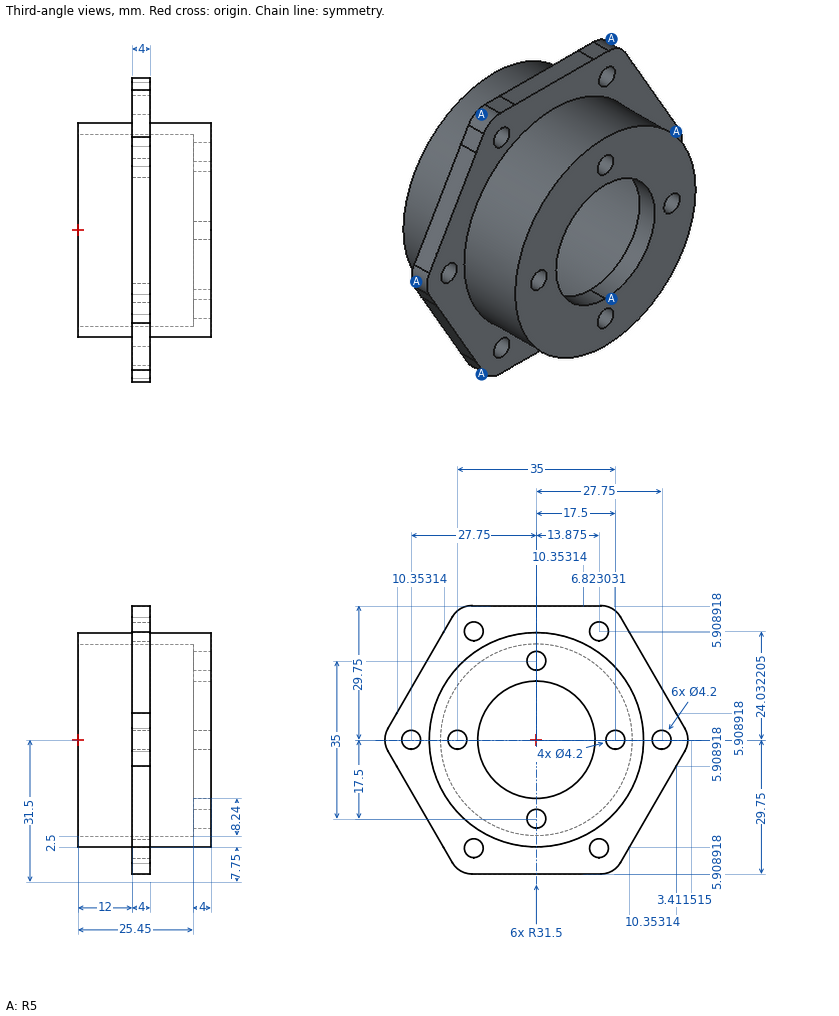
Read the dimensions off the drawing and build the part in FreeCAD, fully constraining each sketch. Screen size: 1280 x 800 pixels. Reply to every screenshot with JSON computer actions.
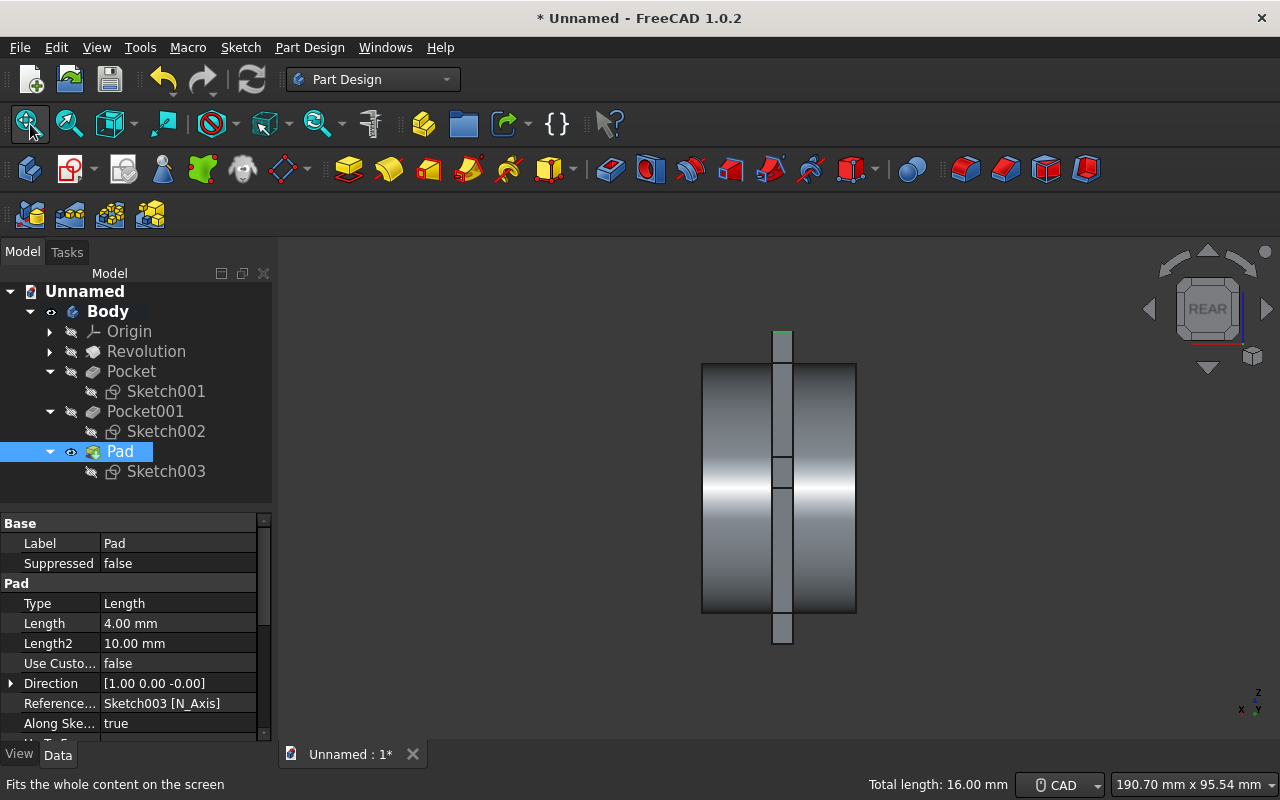
{"action": "left_click", "coordinate": [783, 487], "text": "ctrl"}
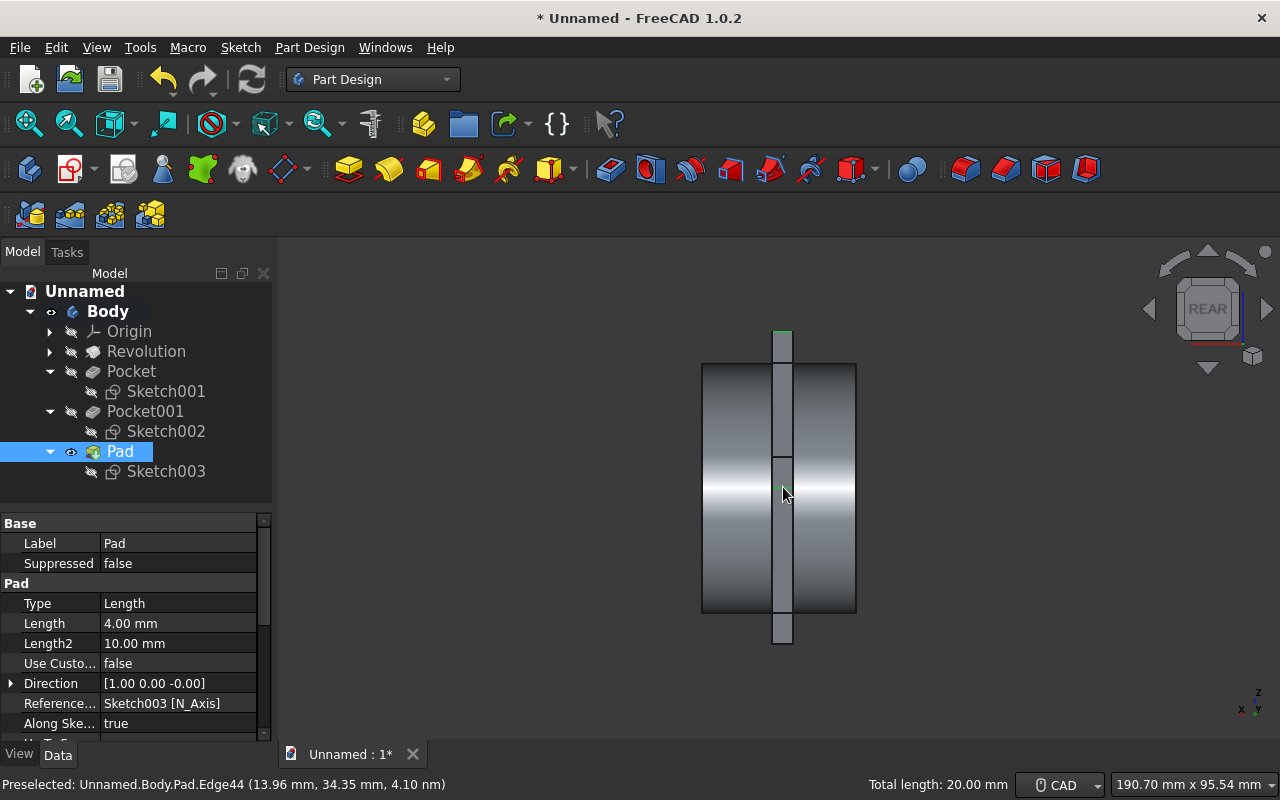
{"action": "scroll", "coordinate": [783, 643], "scroll_direction": "up", "scroll_amount": 4}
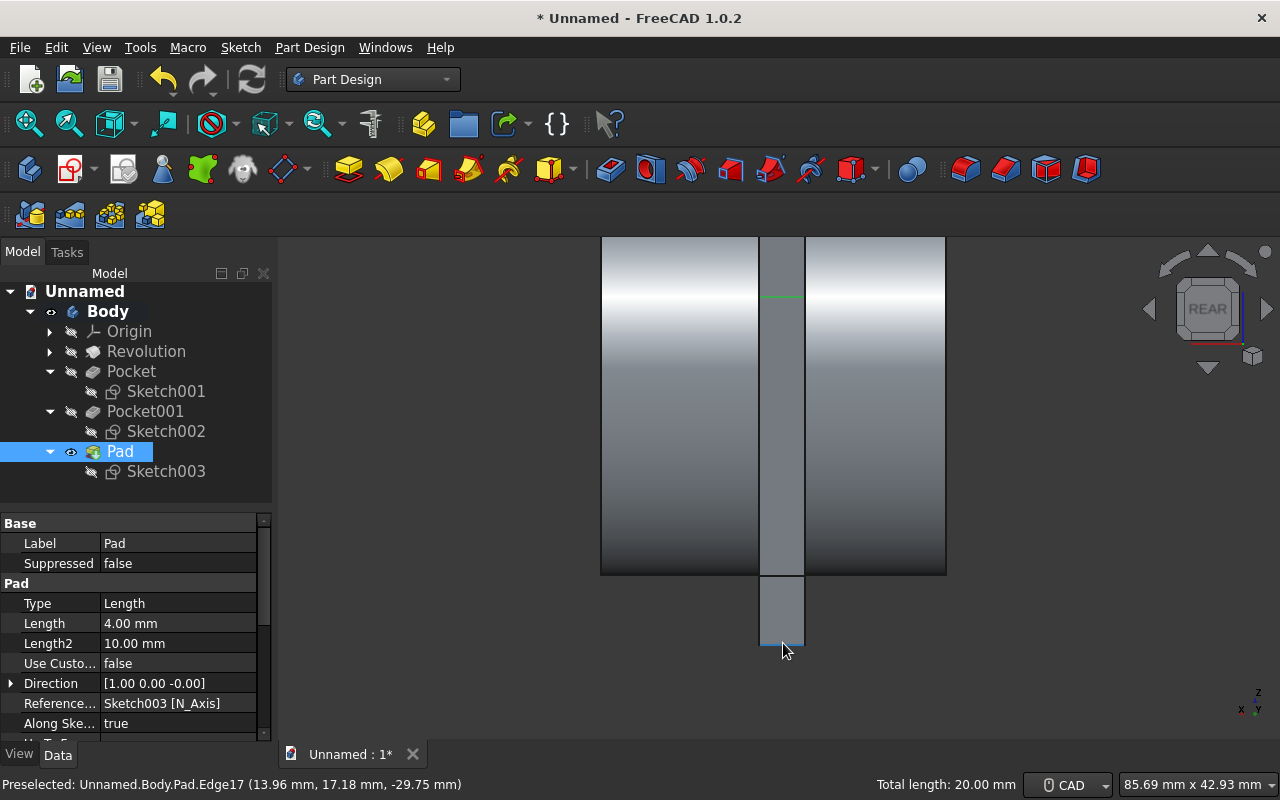
{"action": "key", "text": "v f"}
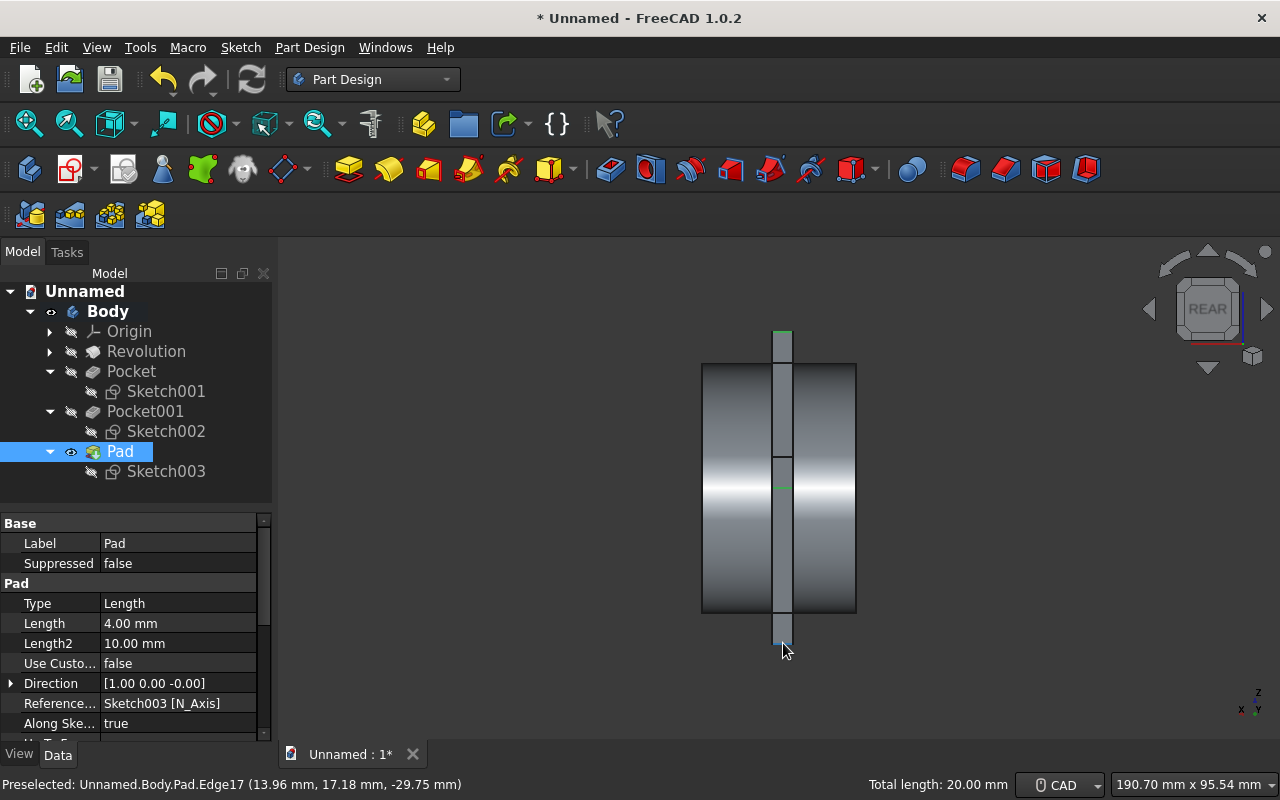
{"action": "key", "text": "6"}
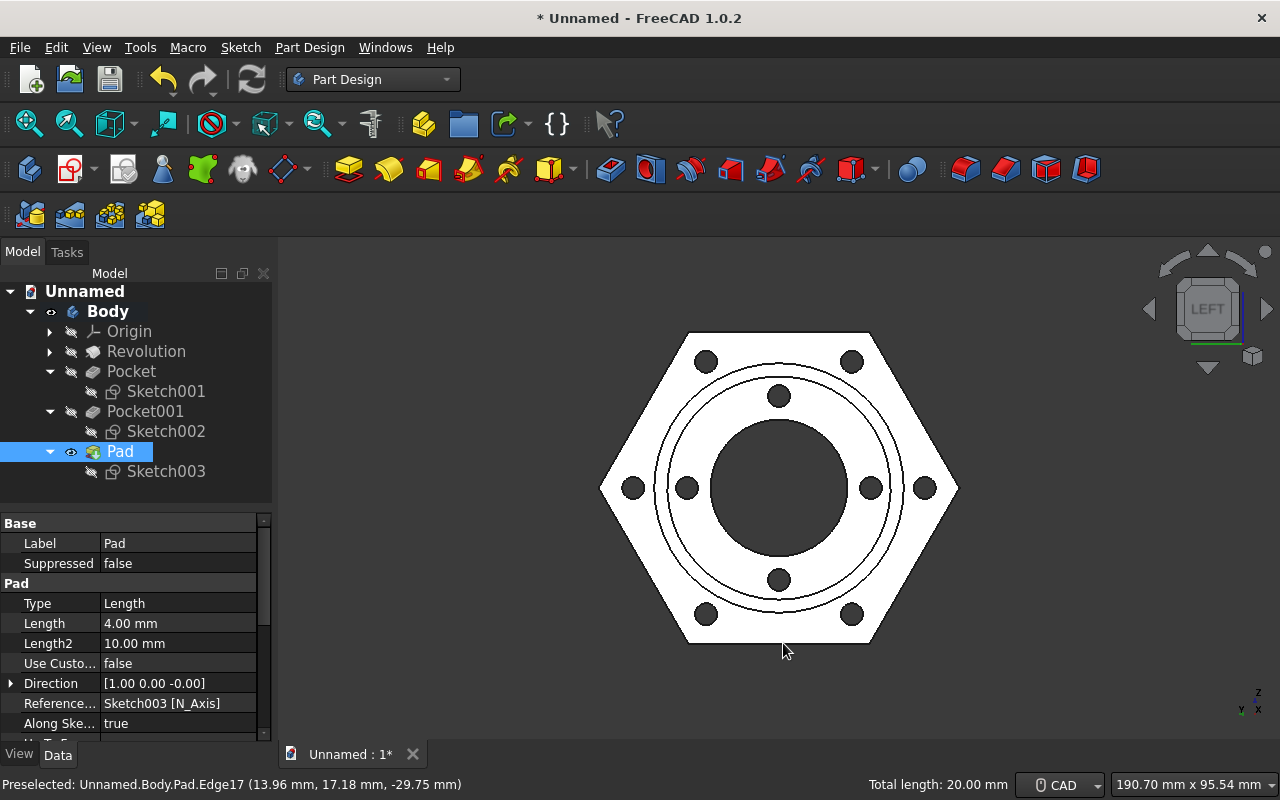
{"action": "scroll", "coordinate": [689, 643], "scroll_direction": "up", "scroll_amount": 4}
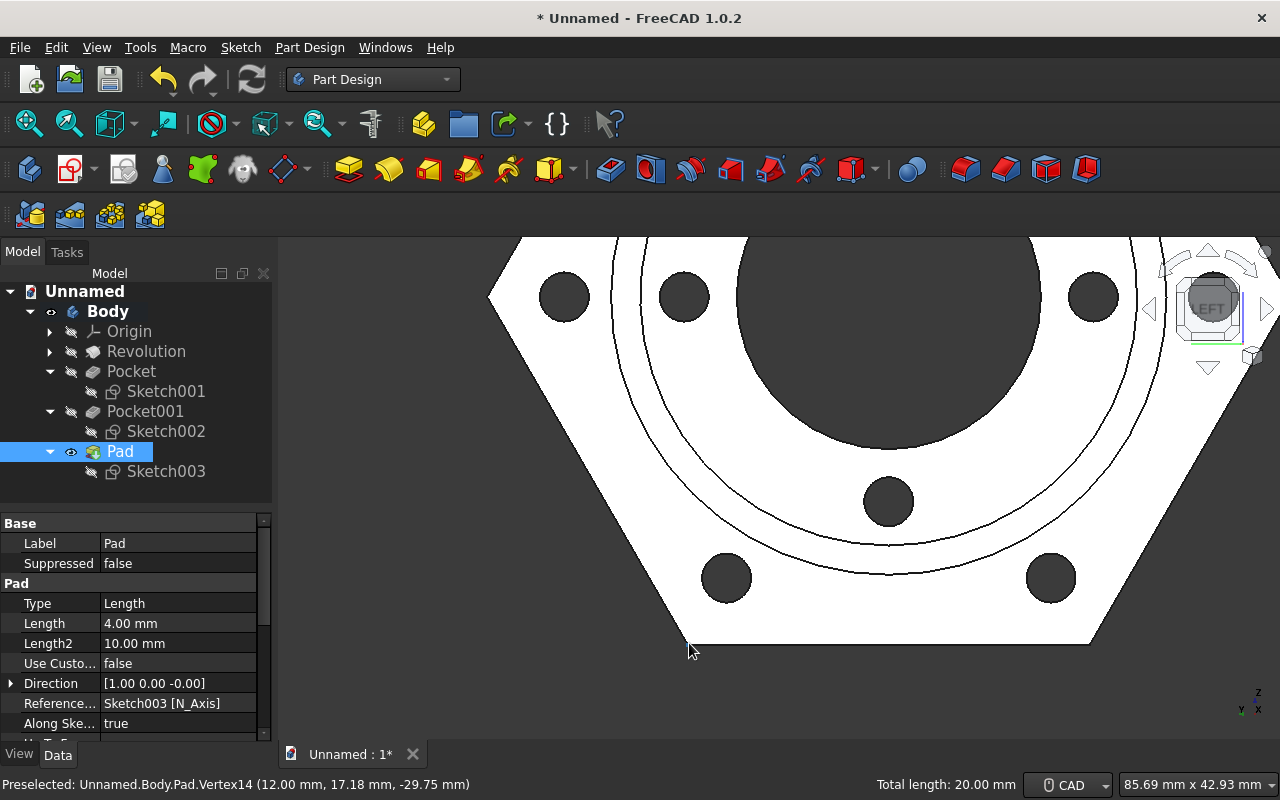
{"action": "key", "text": "v f"}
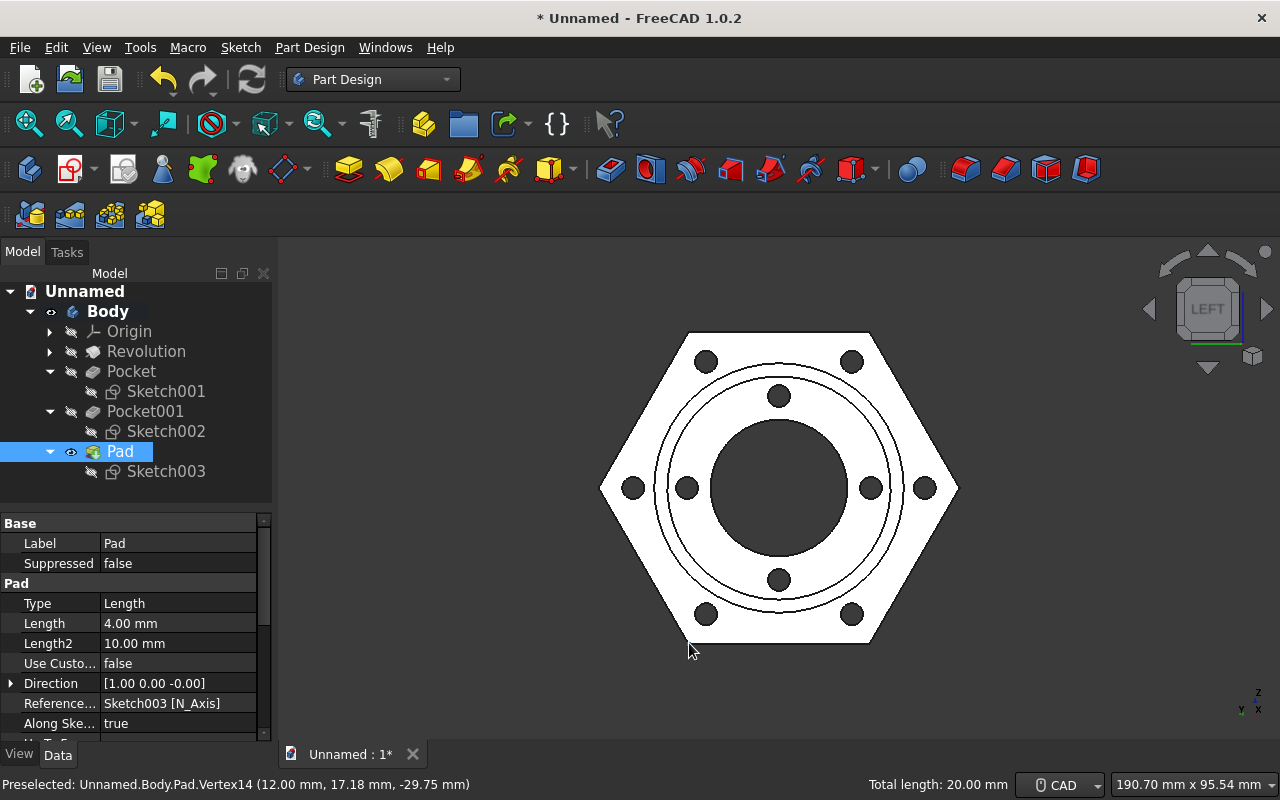
{"action": "key", "text": "v 3"}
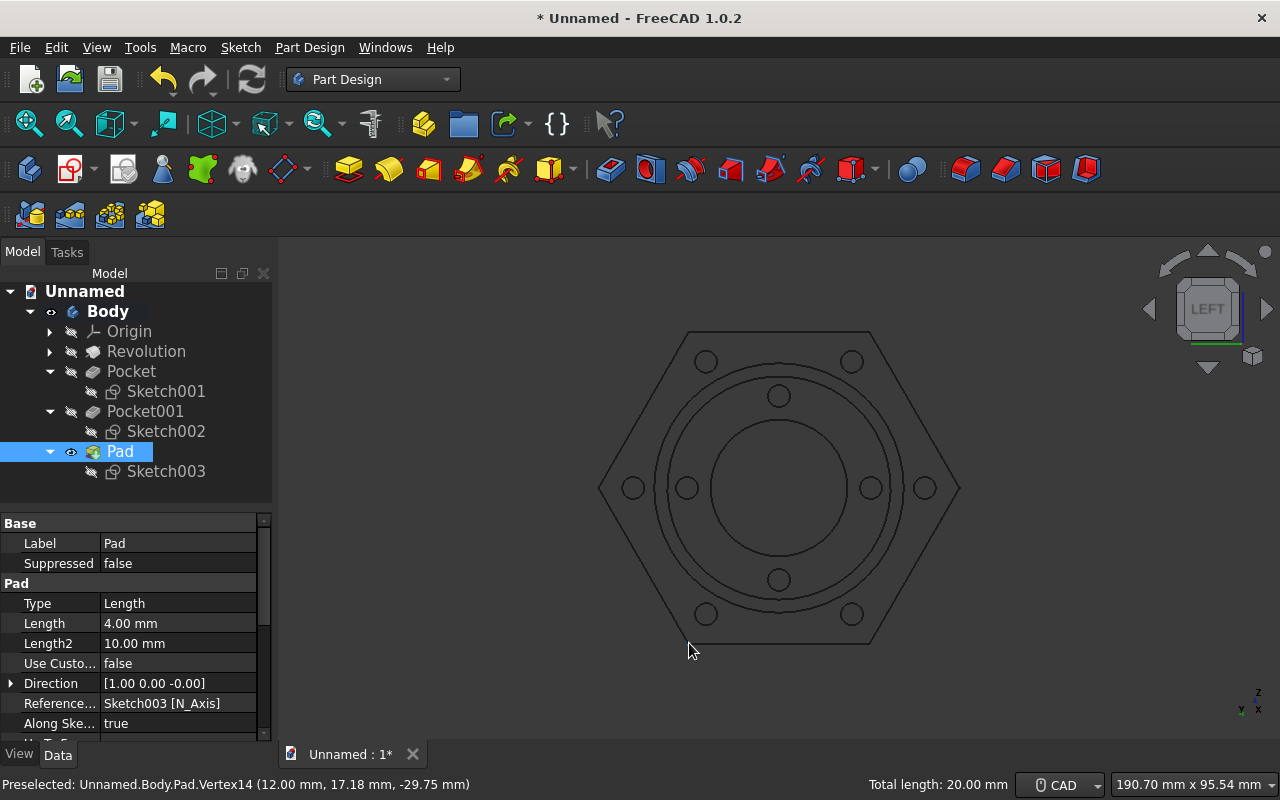
{"action": "key", "text": "0"}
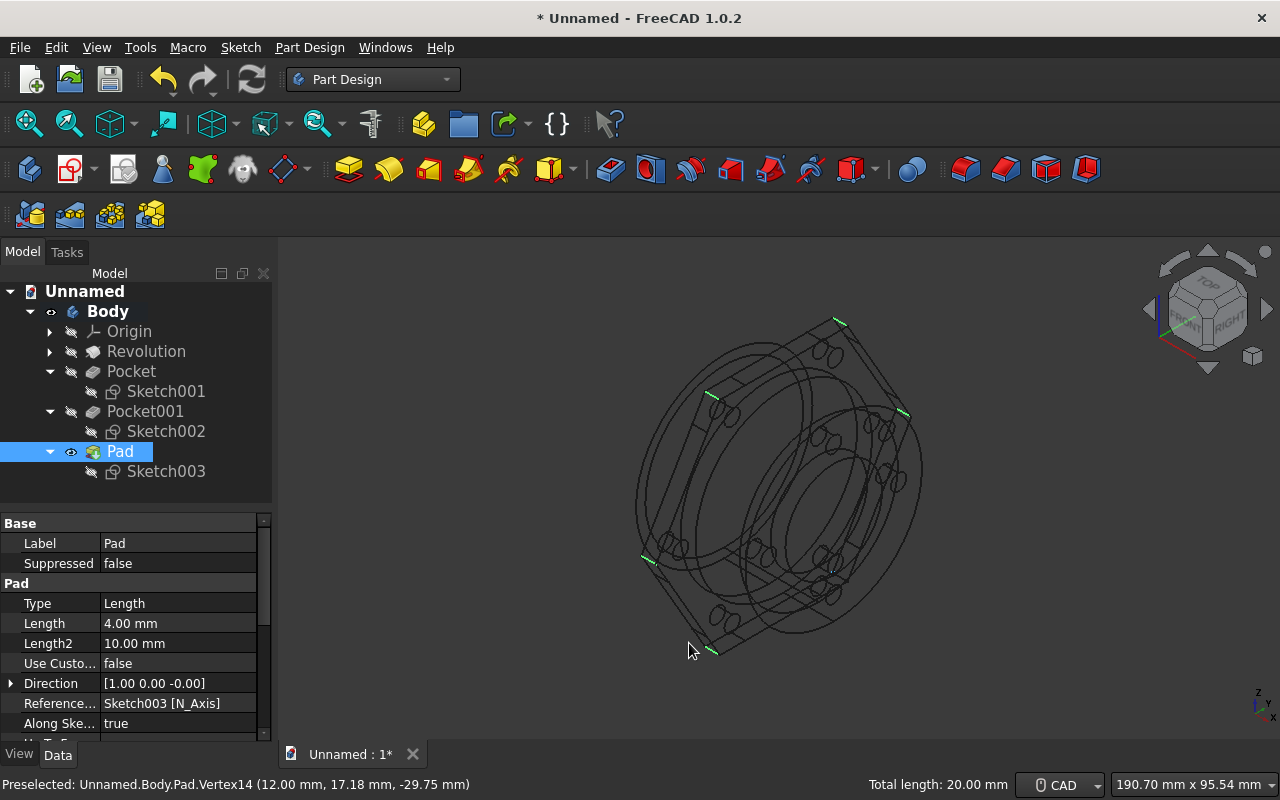
{"action": "scroll", "coordinate": [840, 576], "scroll_direction": "up", "scroll_amount": 4}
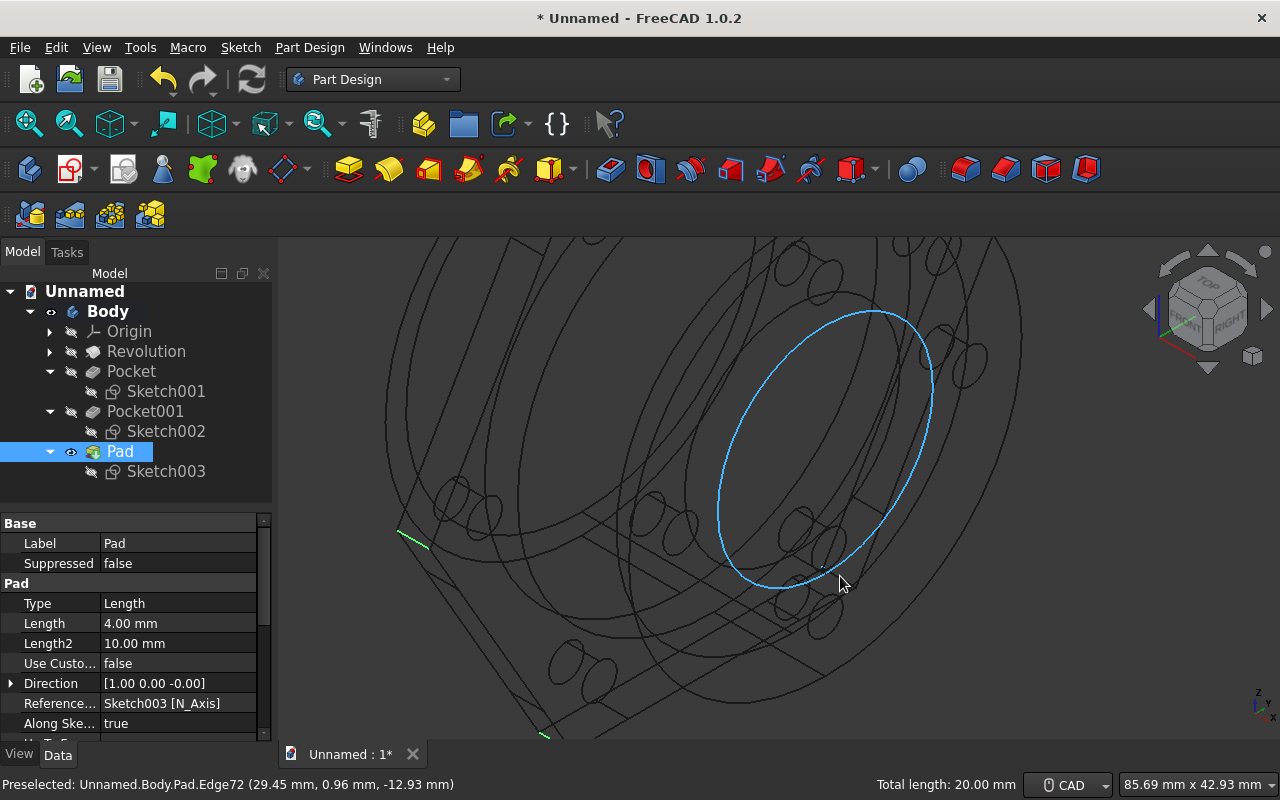
{"action": "left_click", "coordinate": [840, 577], "text": "ctrl"}